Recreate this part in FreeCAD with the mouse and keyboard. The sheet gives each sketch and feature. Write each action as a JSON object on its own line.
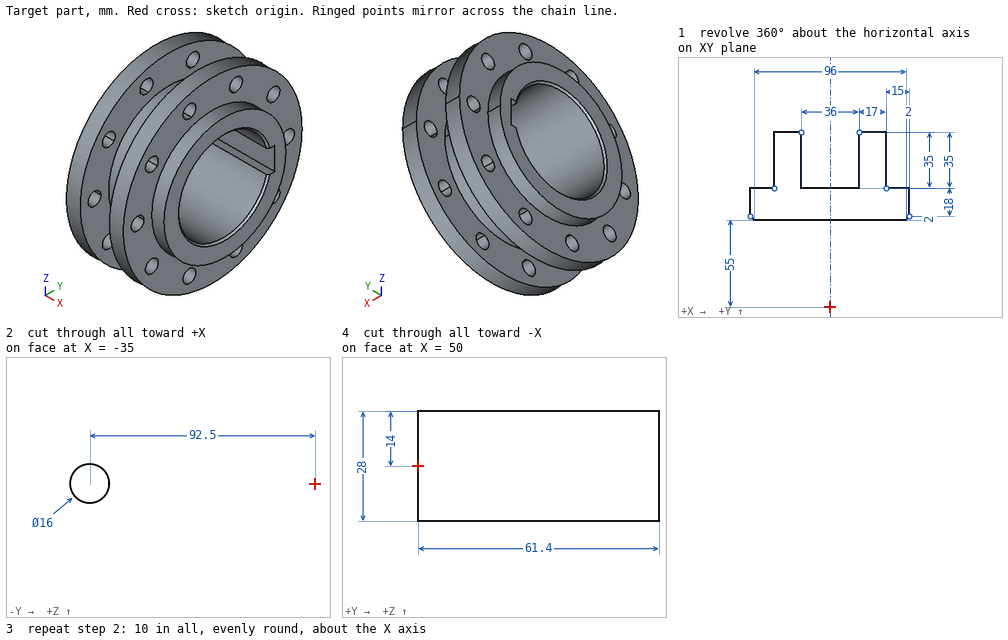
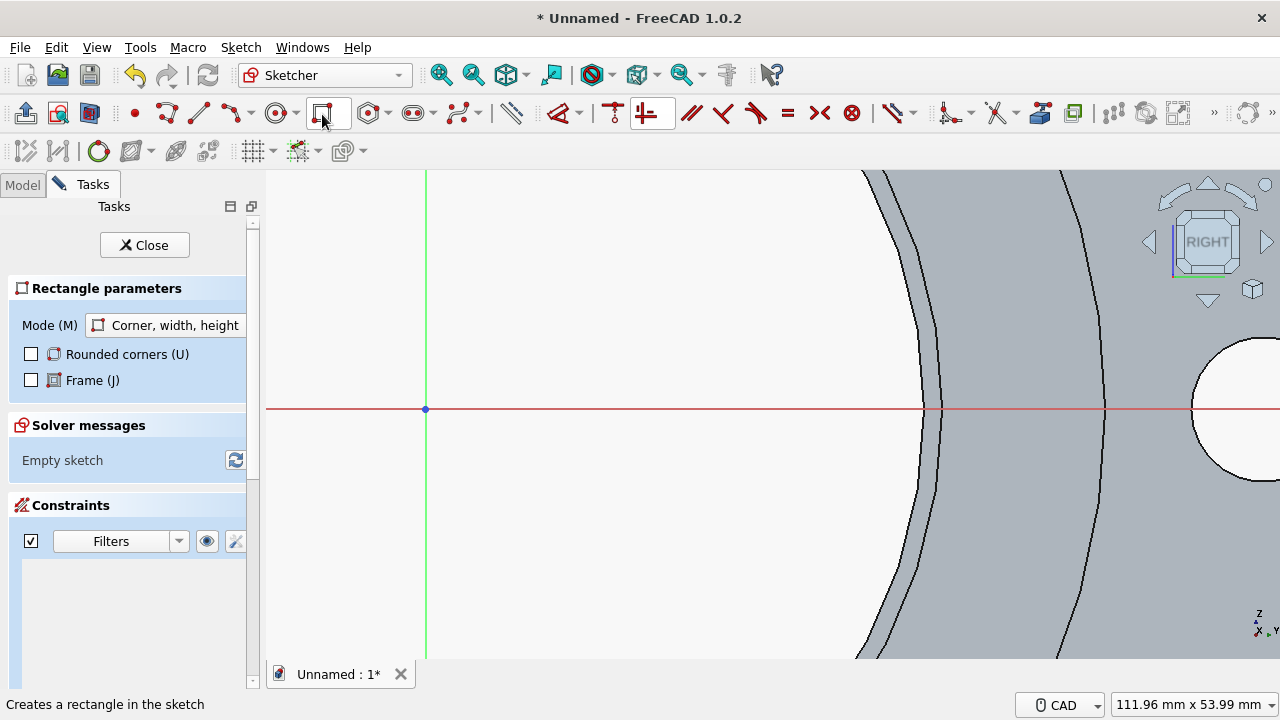
{"action": "left_click", "coordinate": [426, 283]}
{"action": "left_click", "coordinate": [982, 536]}
{"action": "key", "text": "Escape"}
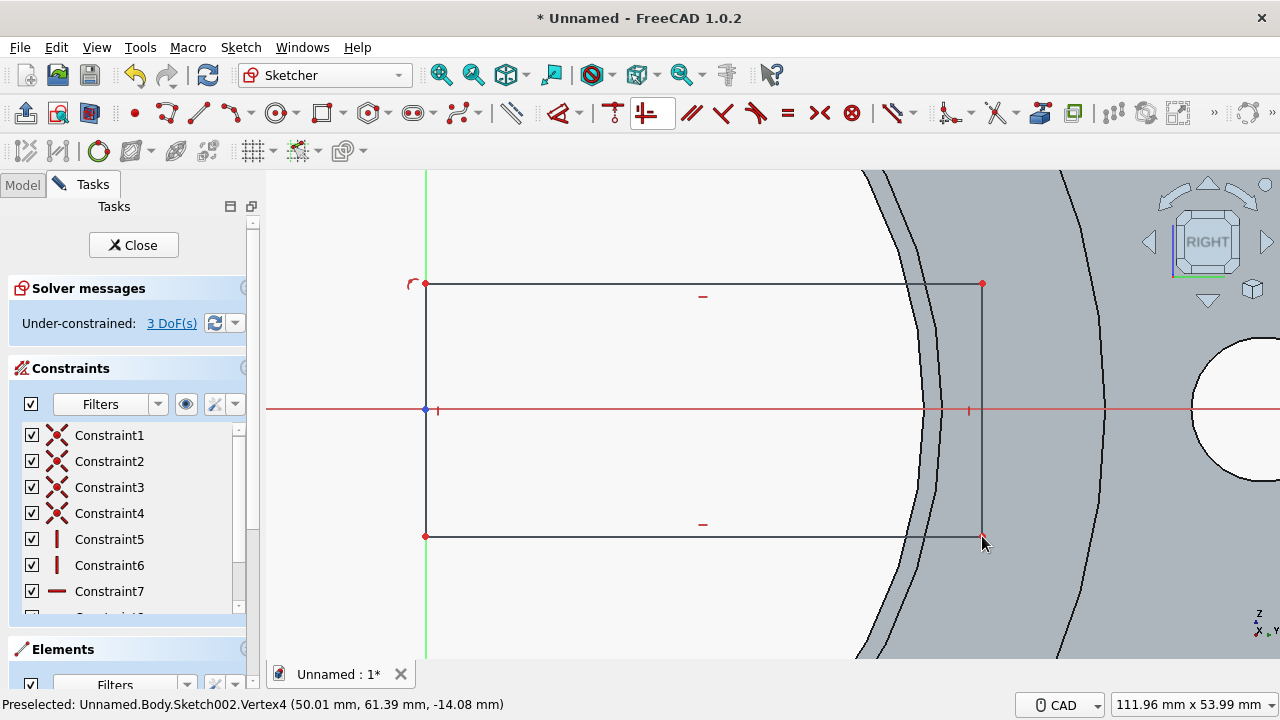
{"action": "left_click", "coordinate": [558, 114]}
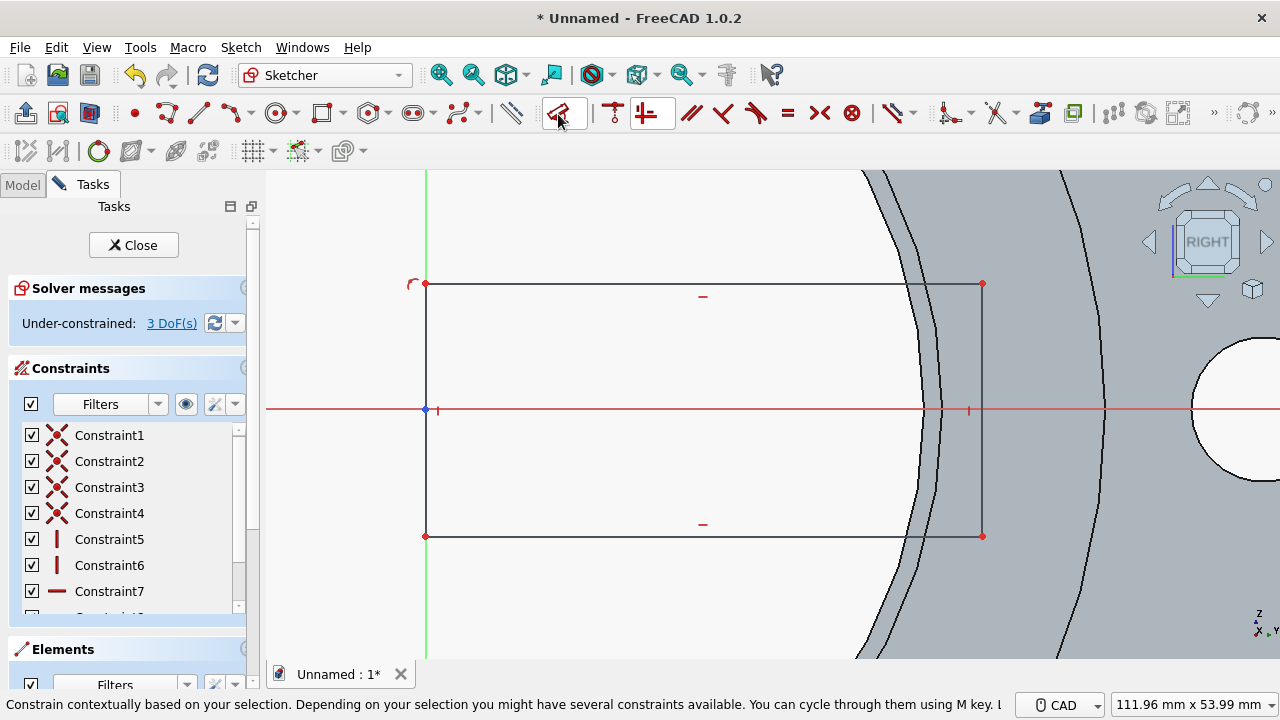
{"action": "left_click", "coordinate": [426, 360]}
{"action": "left_click", "coordinate": [392, 352]}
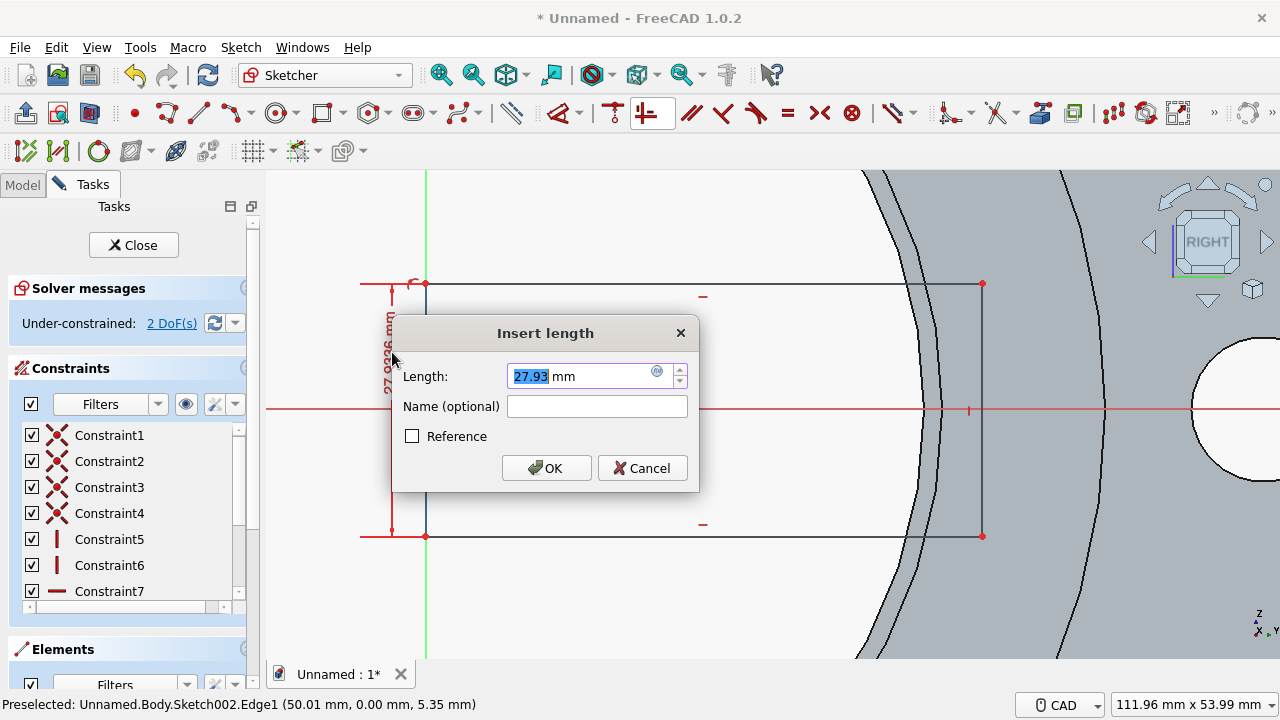
{"action": "type", "text": "28"}
{"action": "key", "text": "Return"}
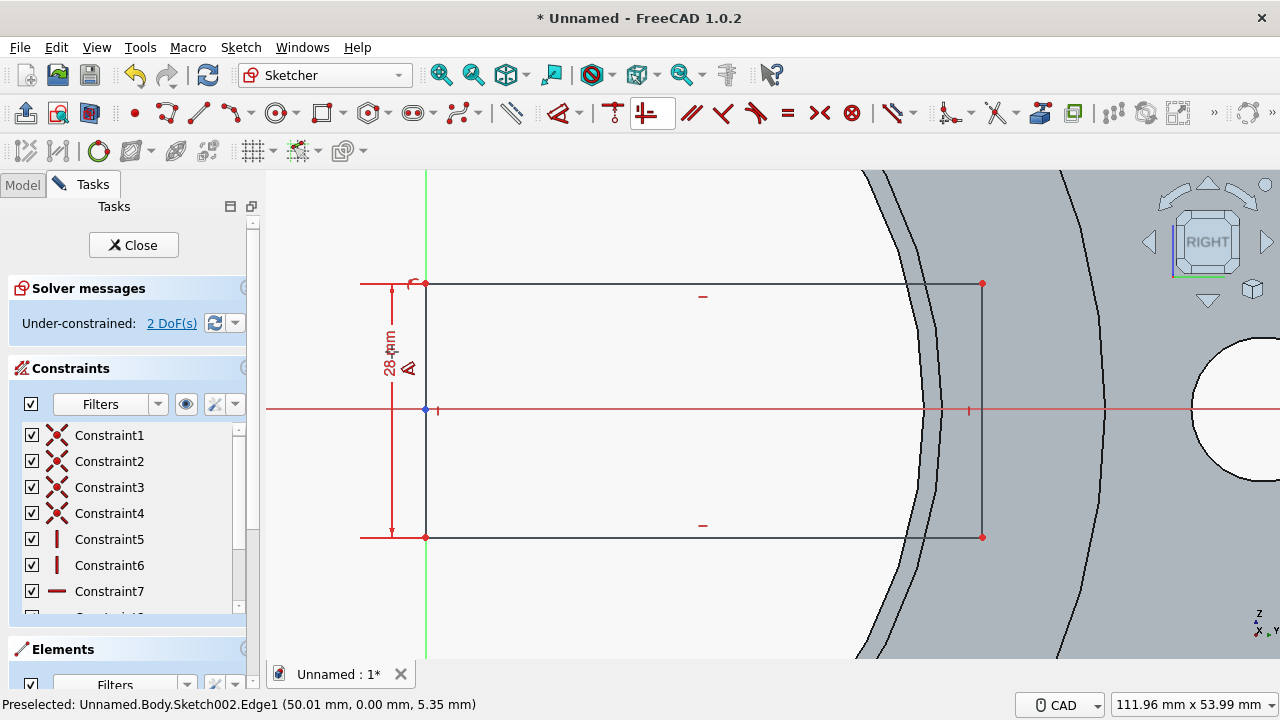
{"action": "left_click", "coordinate": [426, 284]}
{"action": "left_click", "coordinate": [392, 318]}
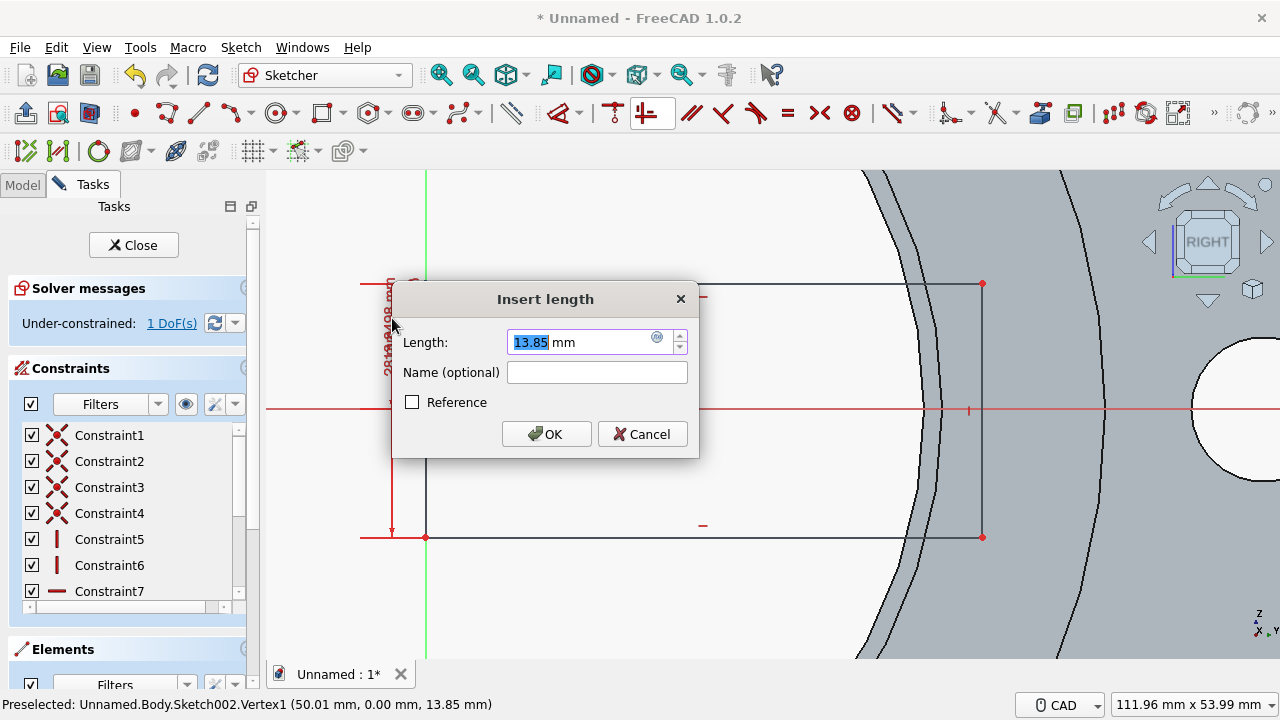
{"action": "type", "text": "14"}
{"action": "key", "text": "Return"}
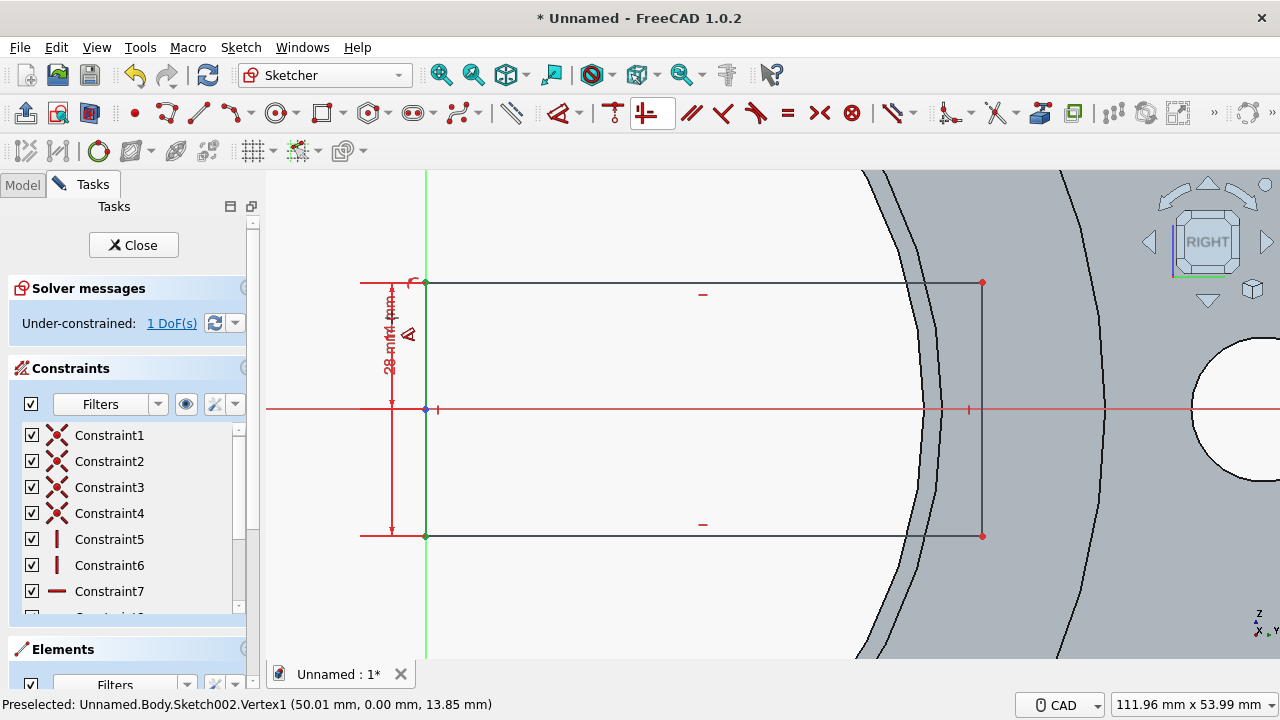
{"action": "left_click", "coordinate": [593, 536]}
{"action": "left_click", "coordinate": [704, 570]}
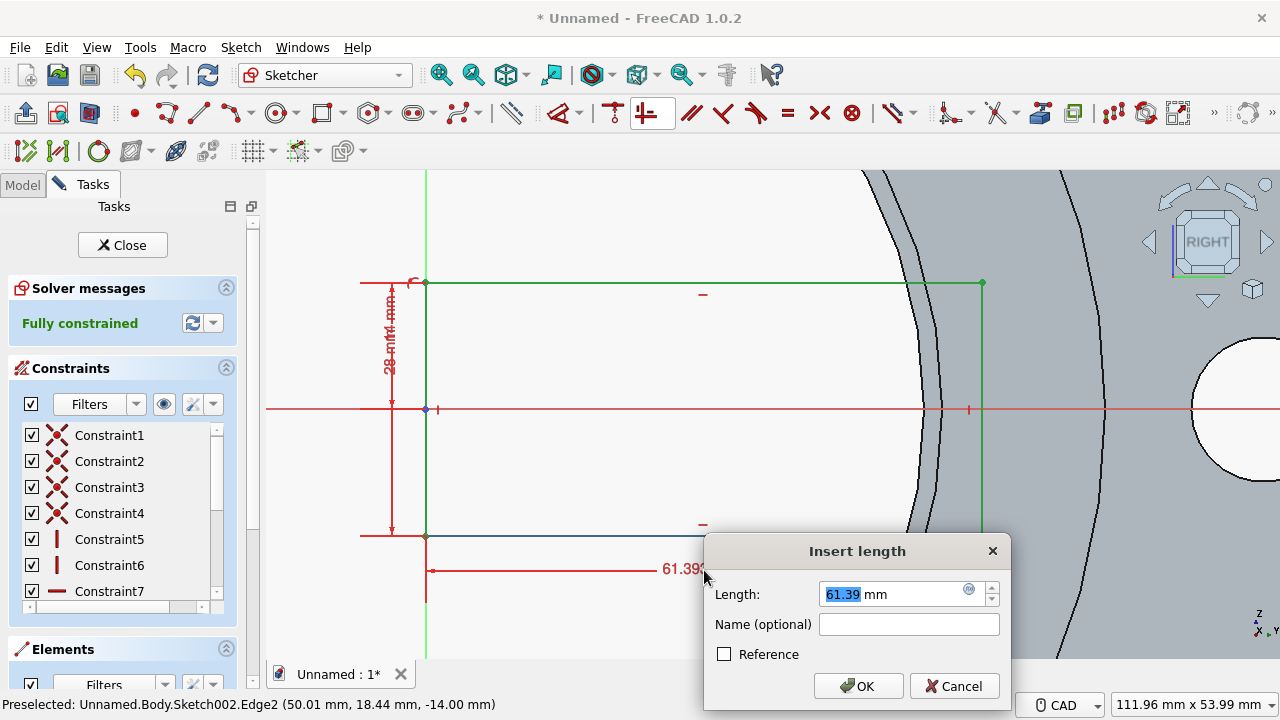
{"action": "type", "text": "61.4"}
{"action": "key", "text": "Return"}
{"action": "key", "text": "Escape"}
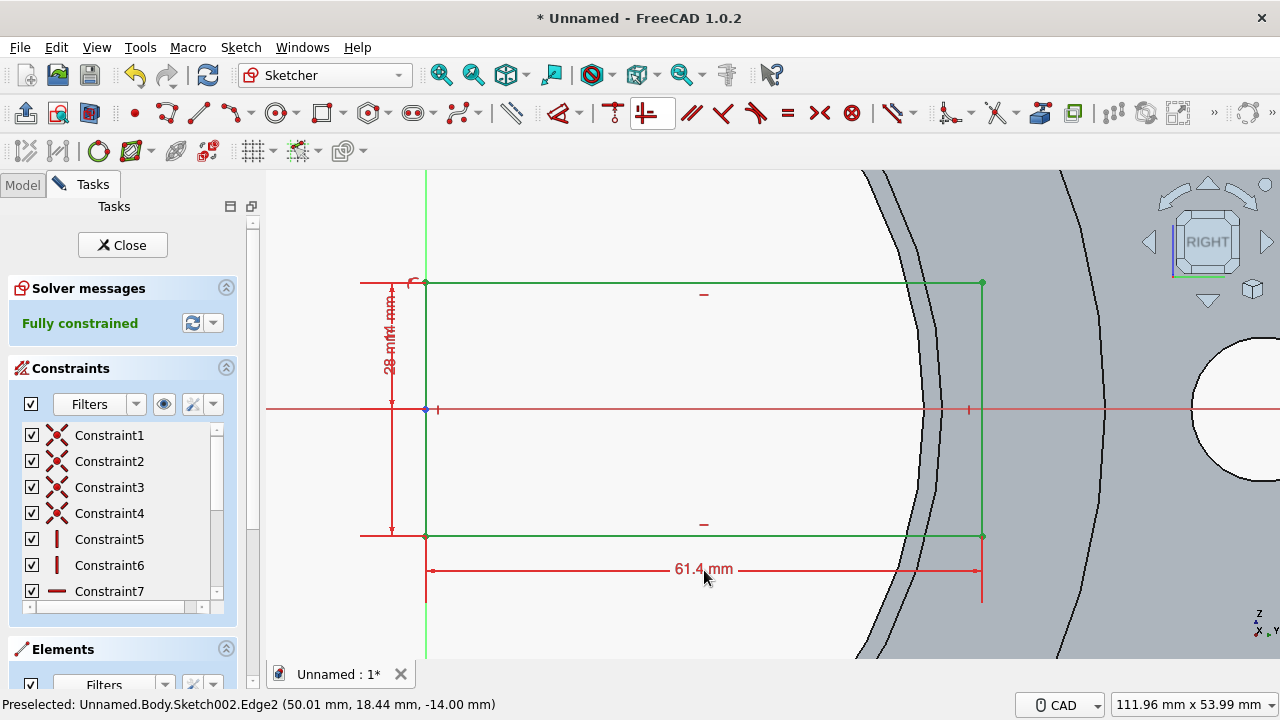
{"action": "left_click", "coordinate": [123, 245]}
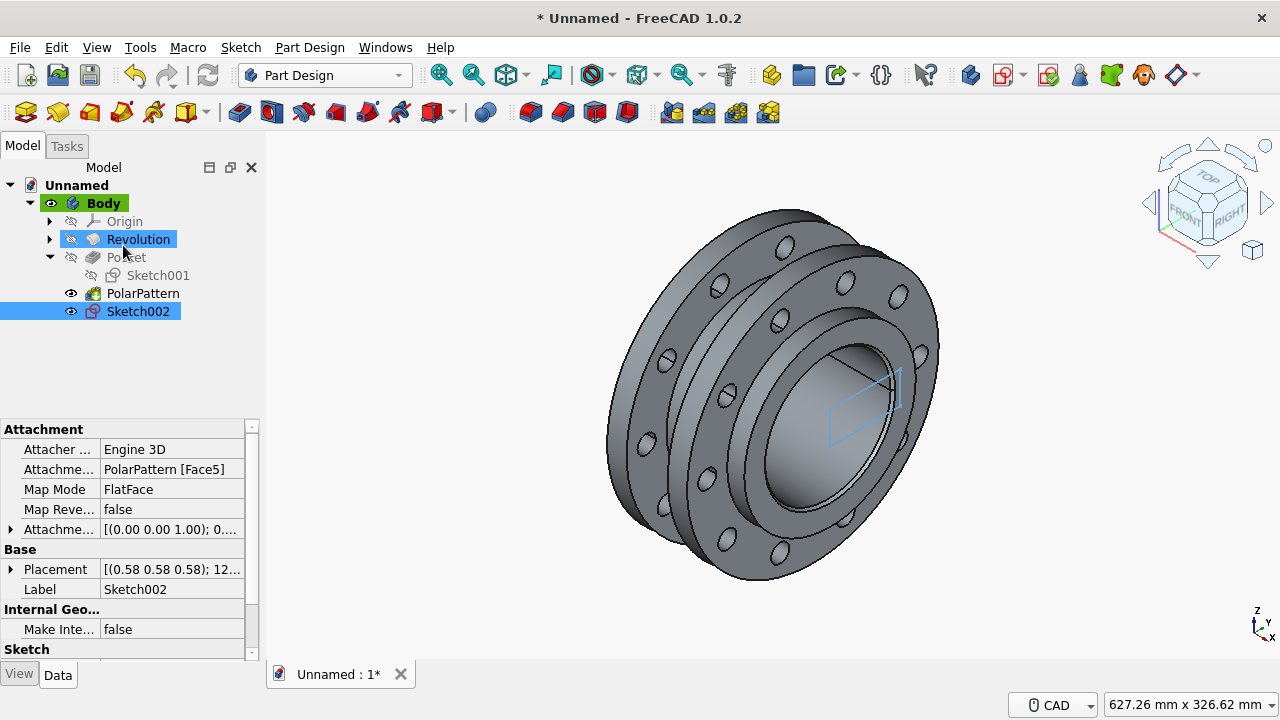
{"action": "left_click", "coordinate": [240, 112]}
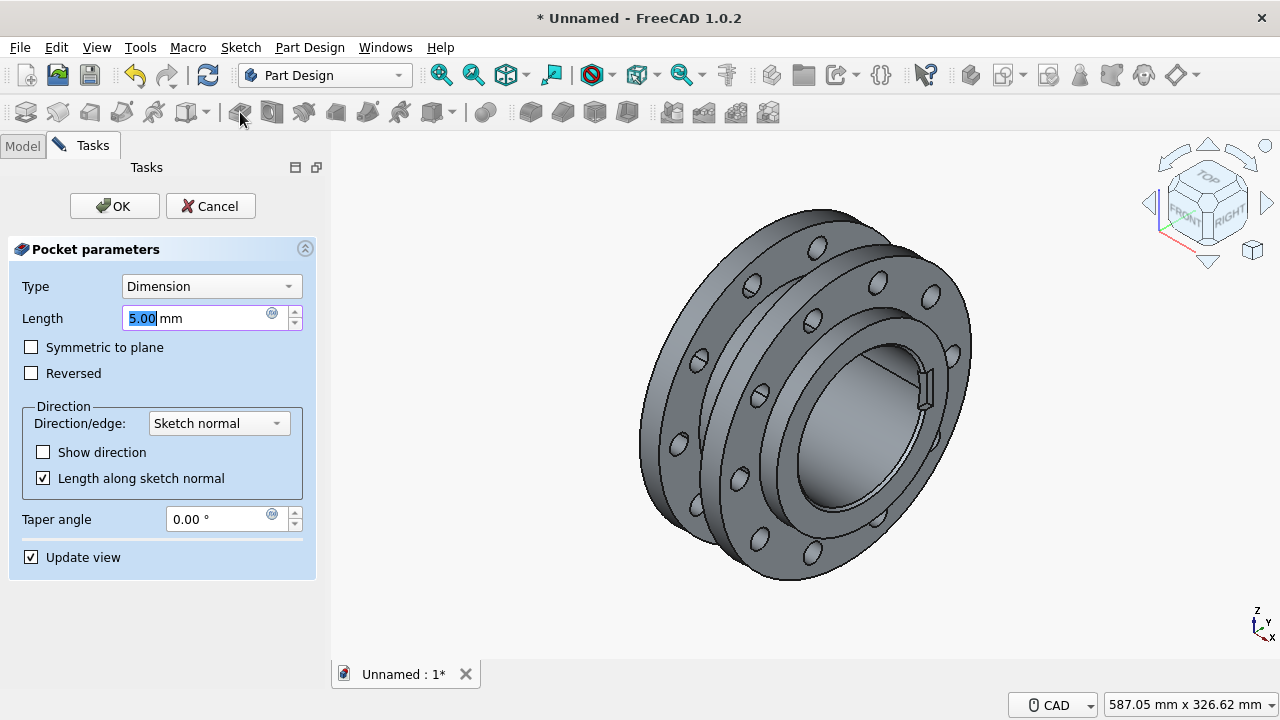
{"action": "left_click", "coordinate": [212, 286]}